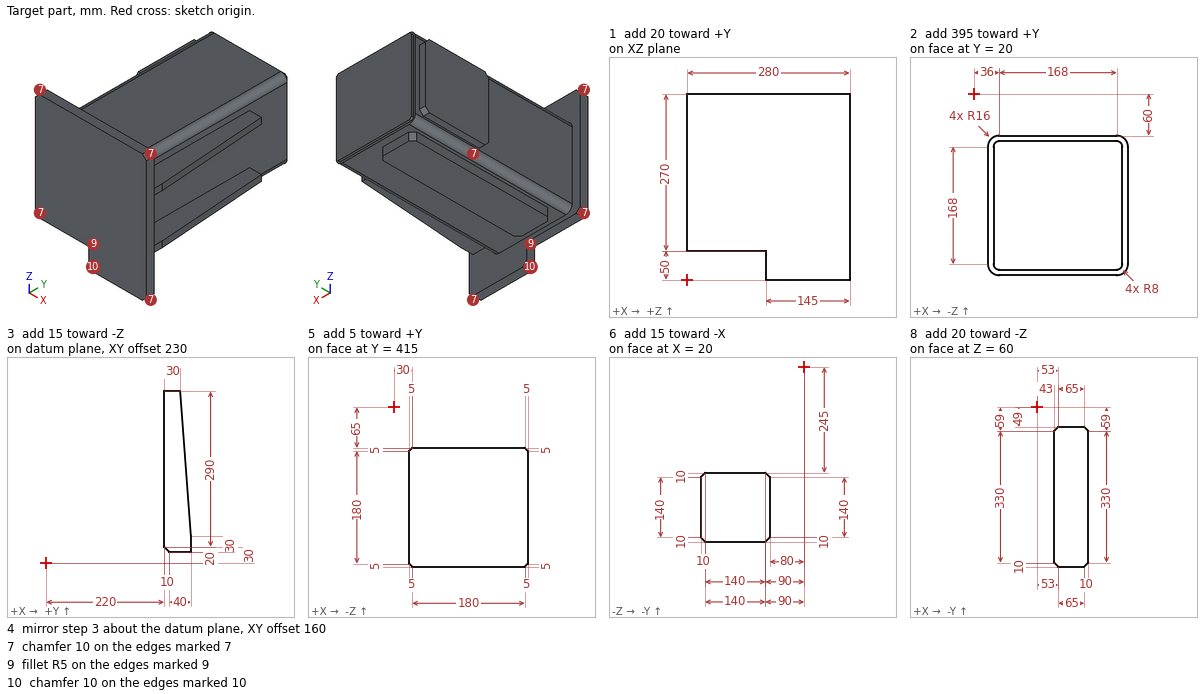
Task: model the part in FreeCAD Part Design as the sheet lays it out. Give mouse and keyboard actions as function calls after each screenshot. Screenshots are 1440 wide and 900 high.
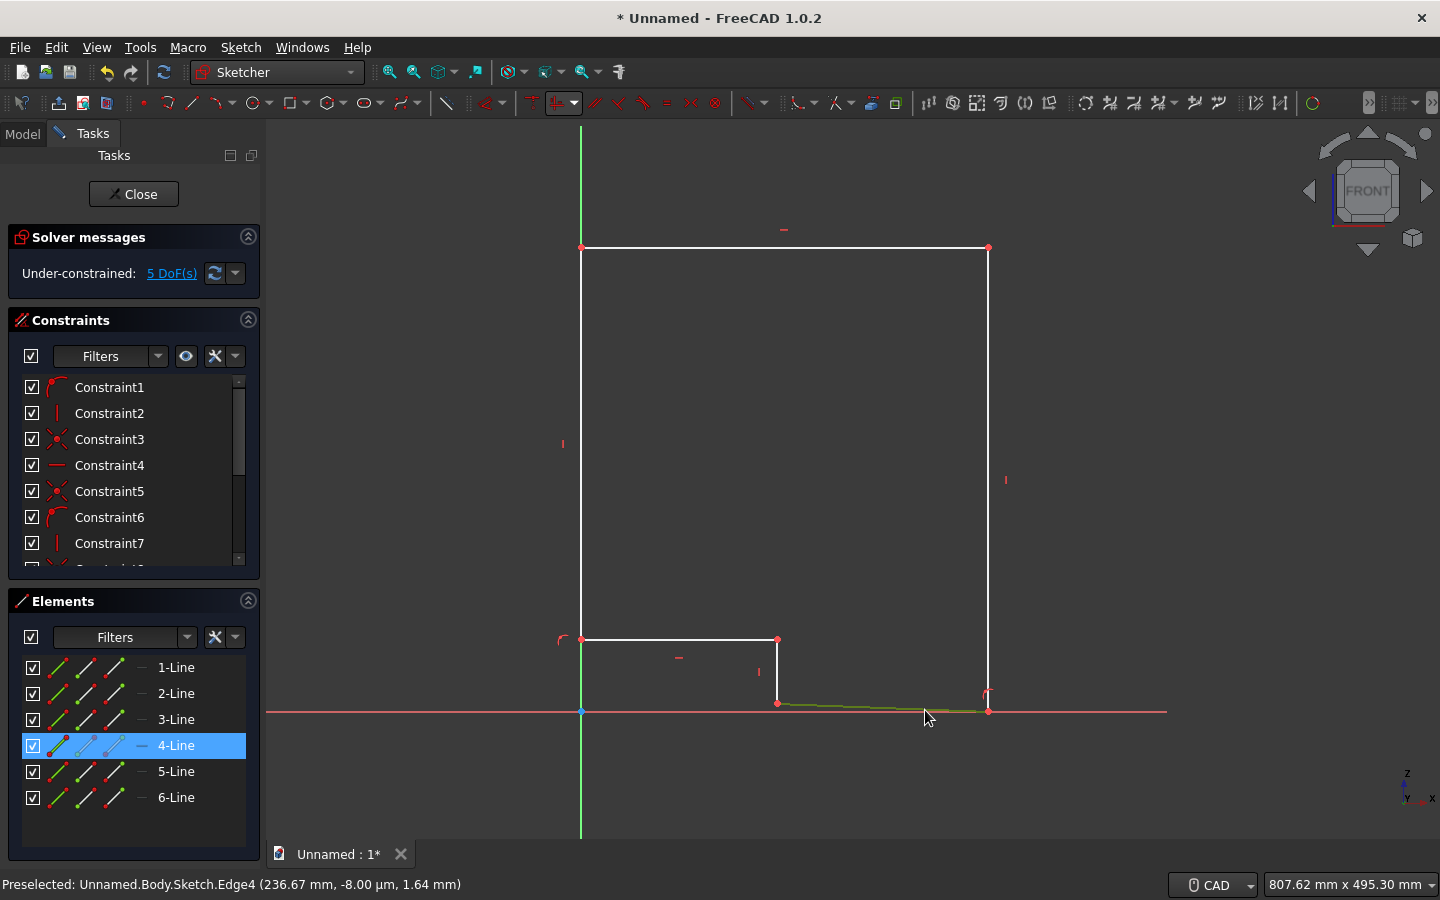
key(h)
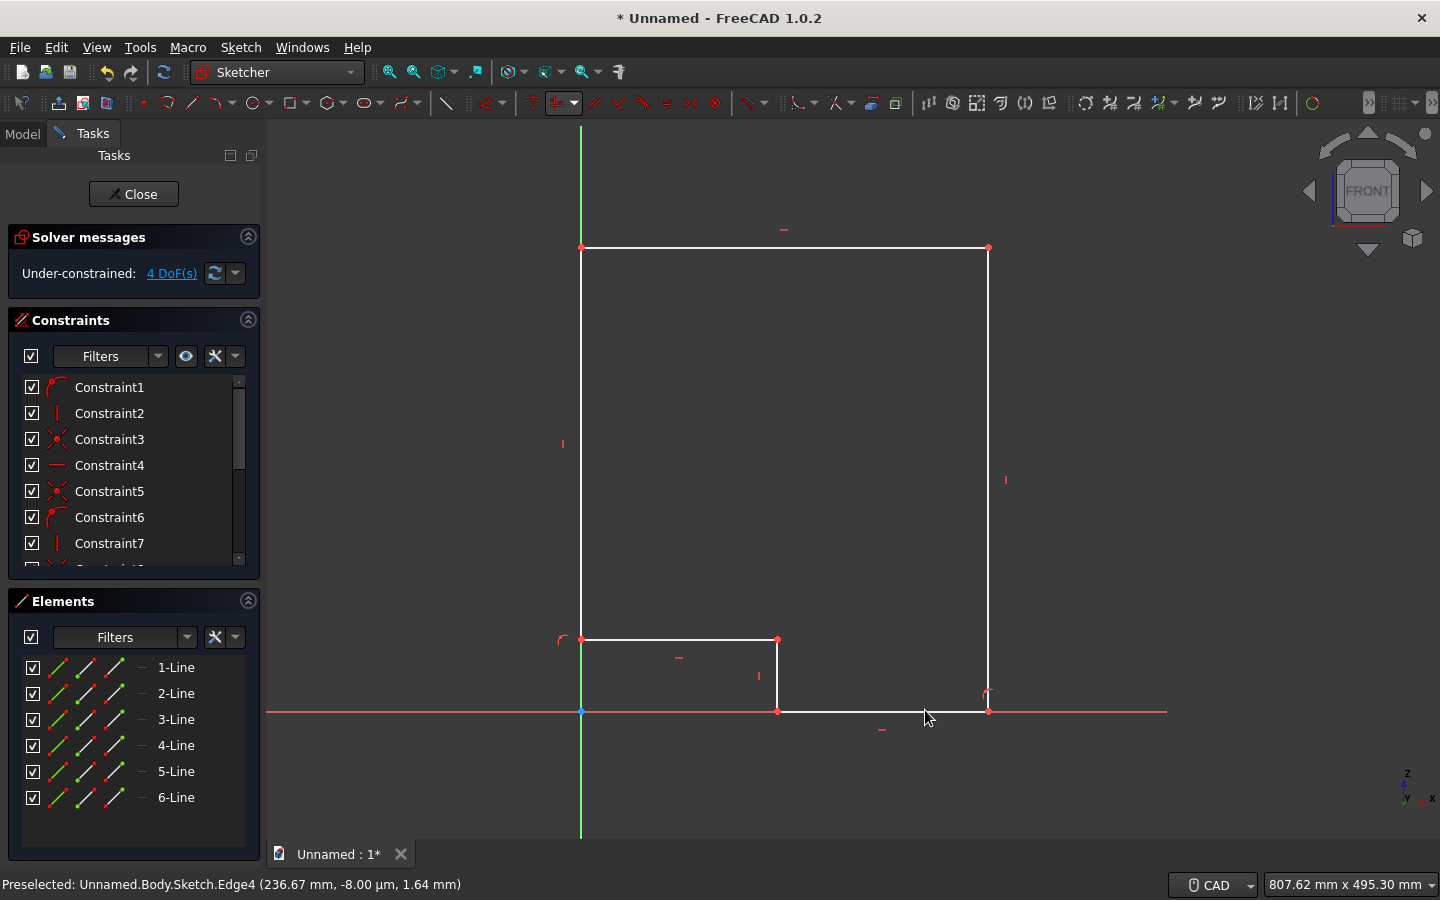
click(486, 104)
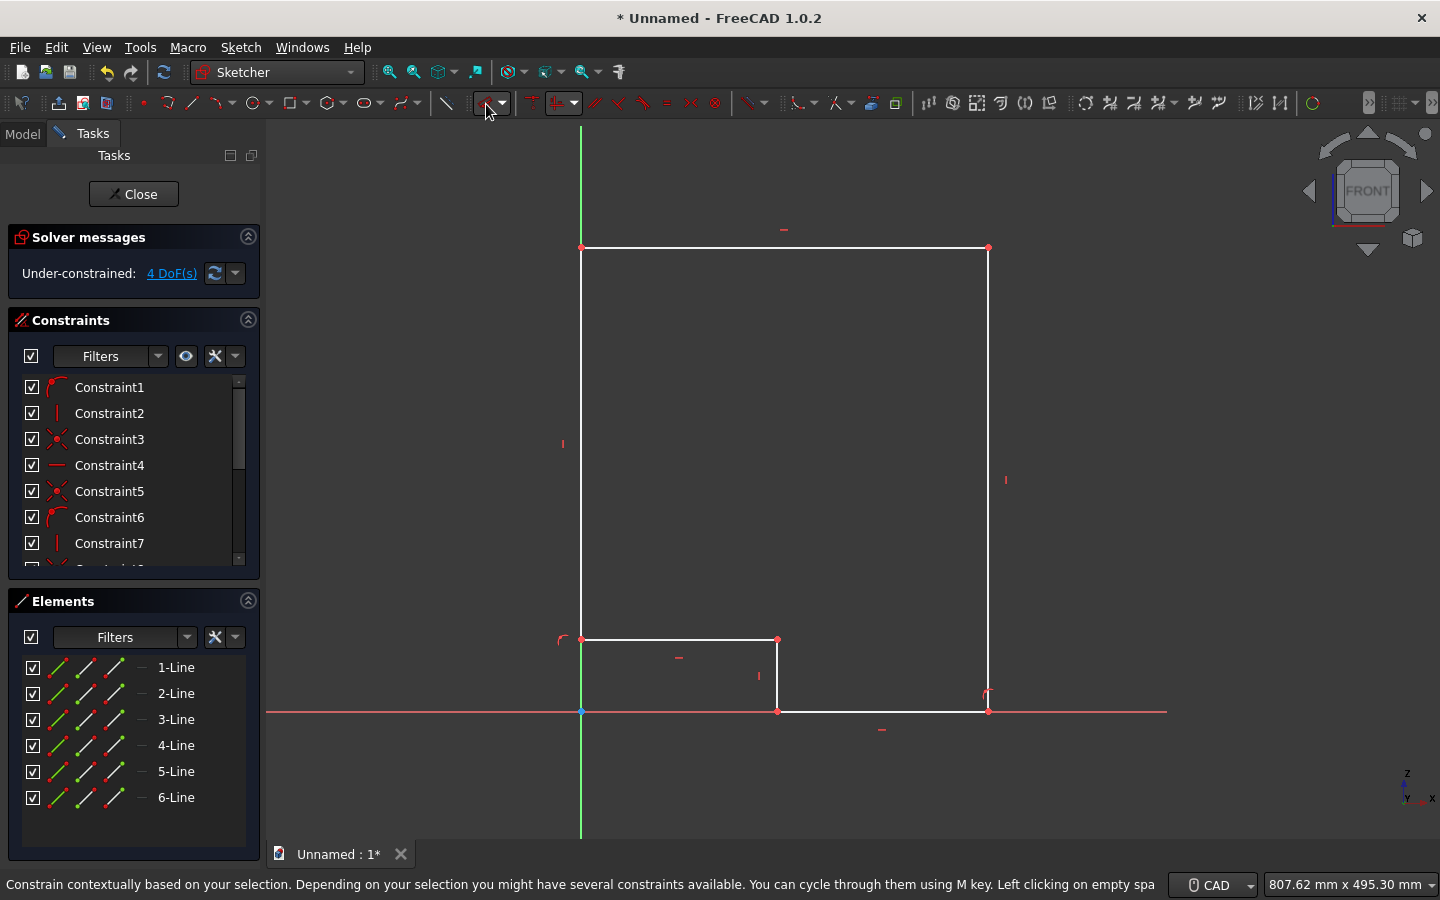
click(777, 690)
click(743, 676)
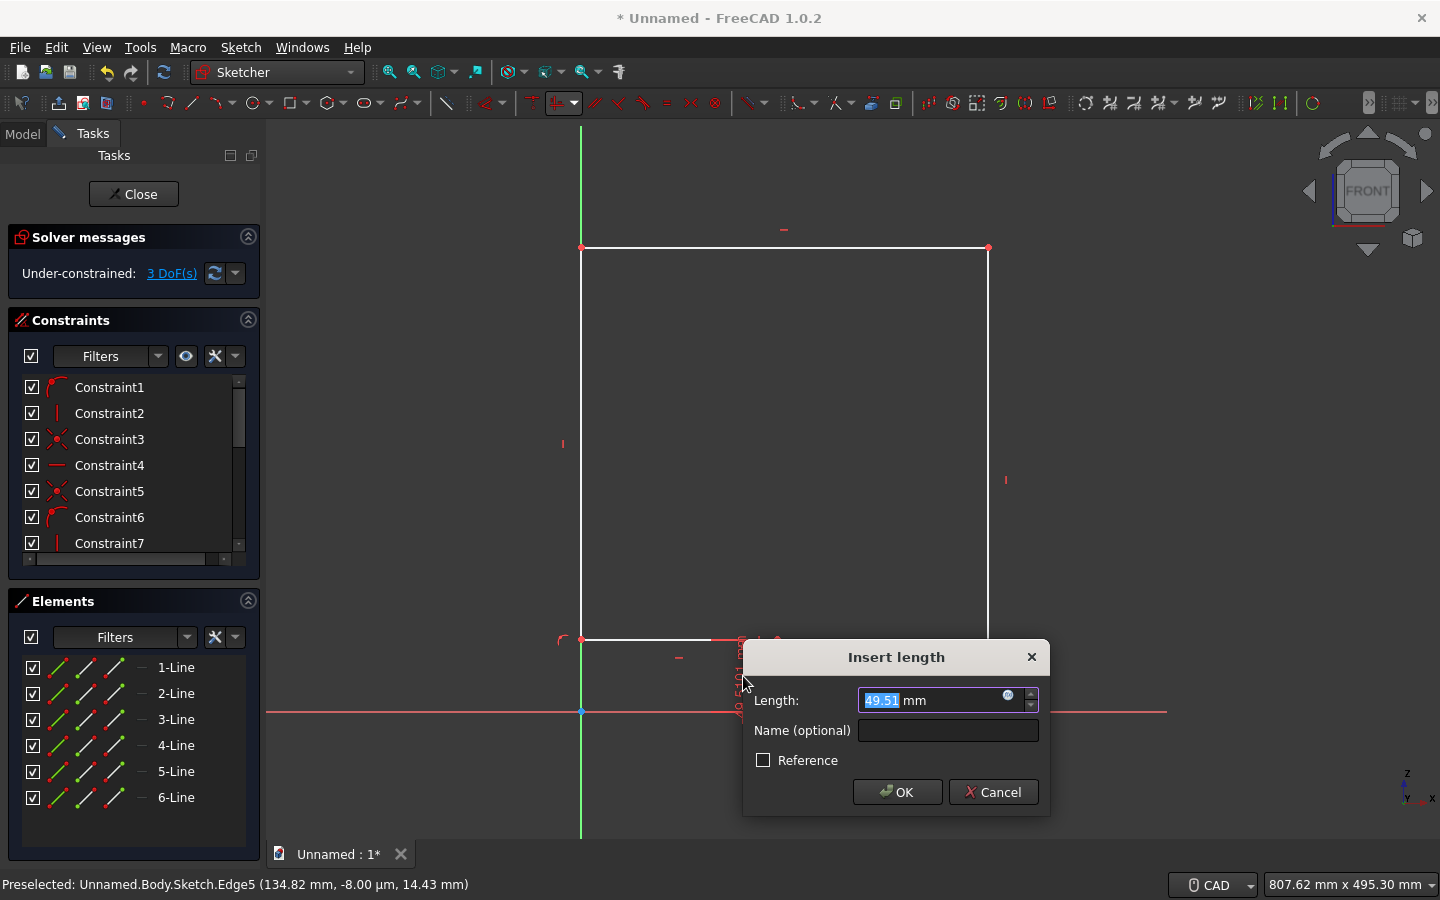
text(50)
key(Return)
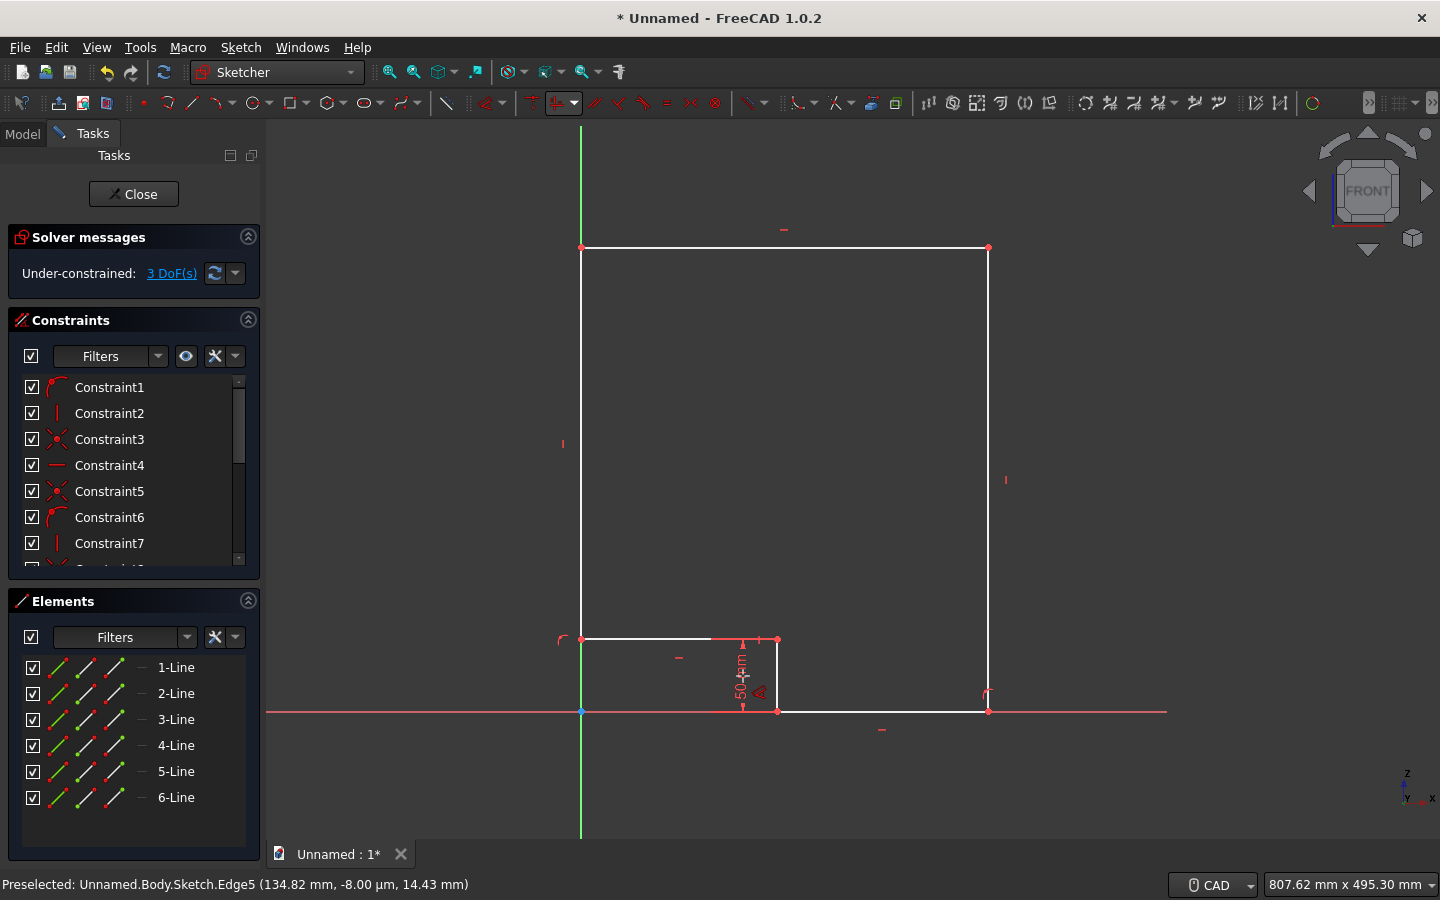
click(581, 522)
click(547, 444)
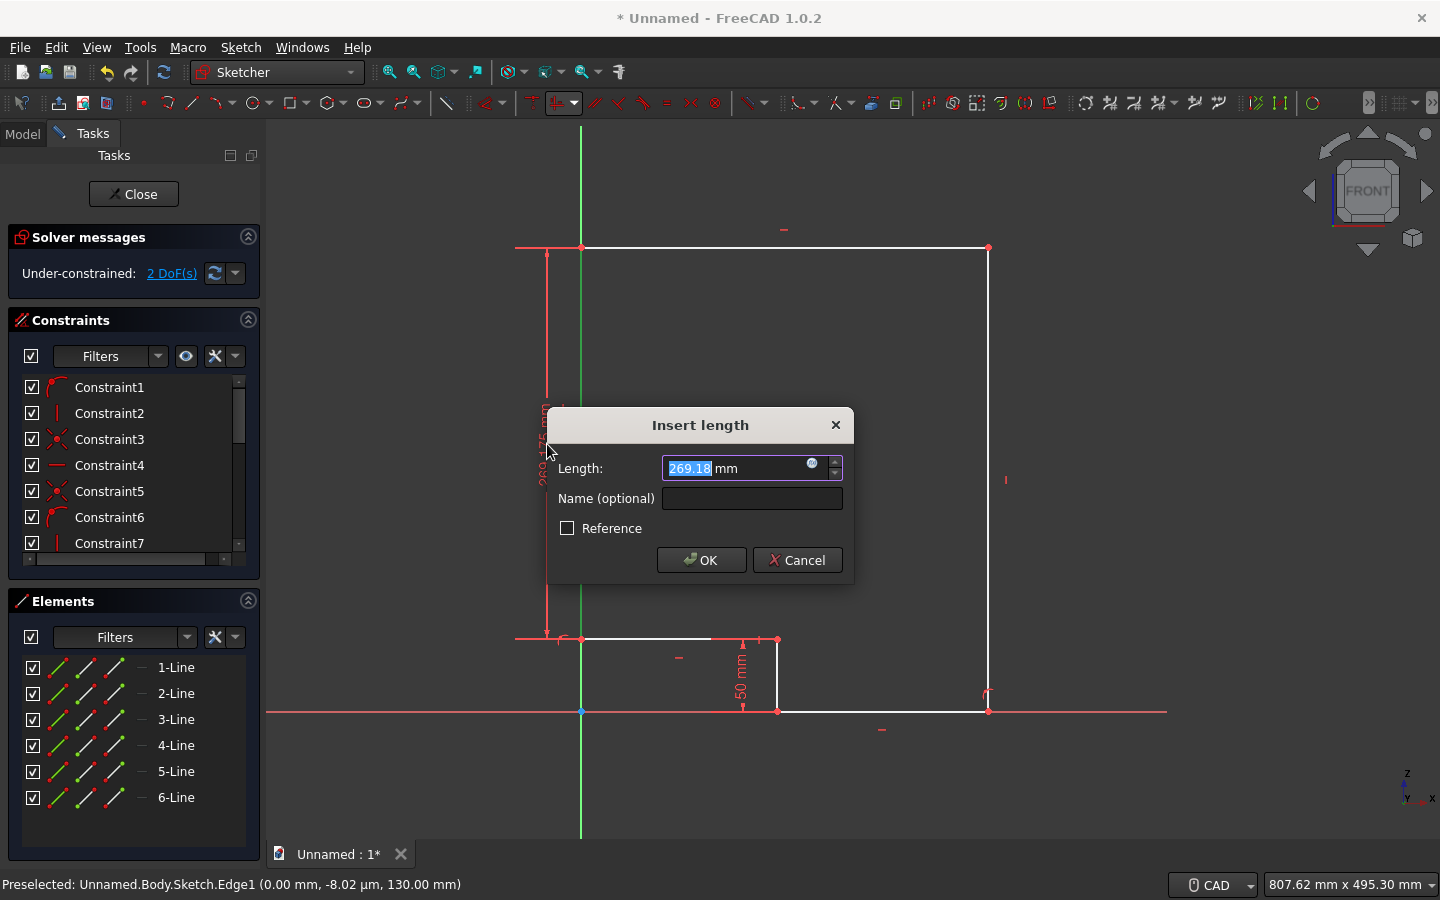
text(270)
key(Return)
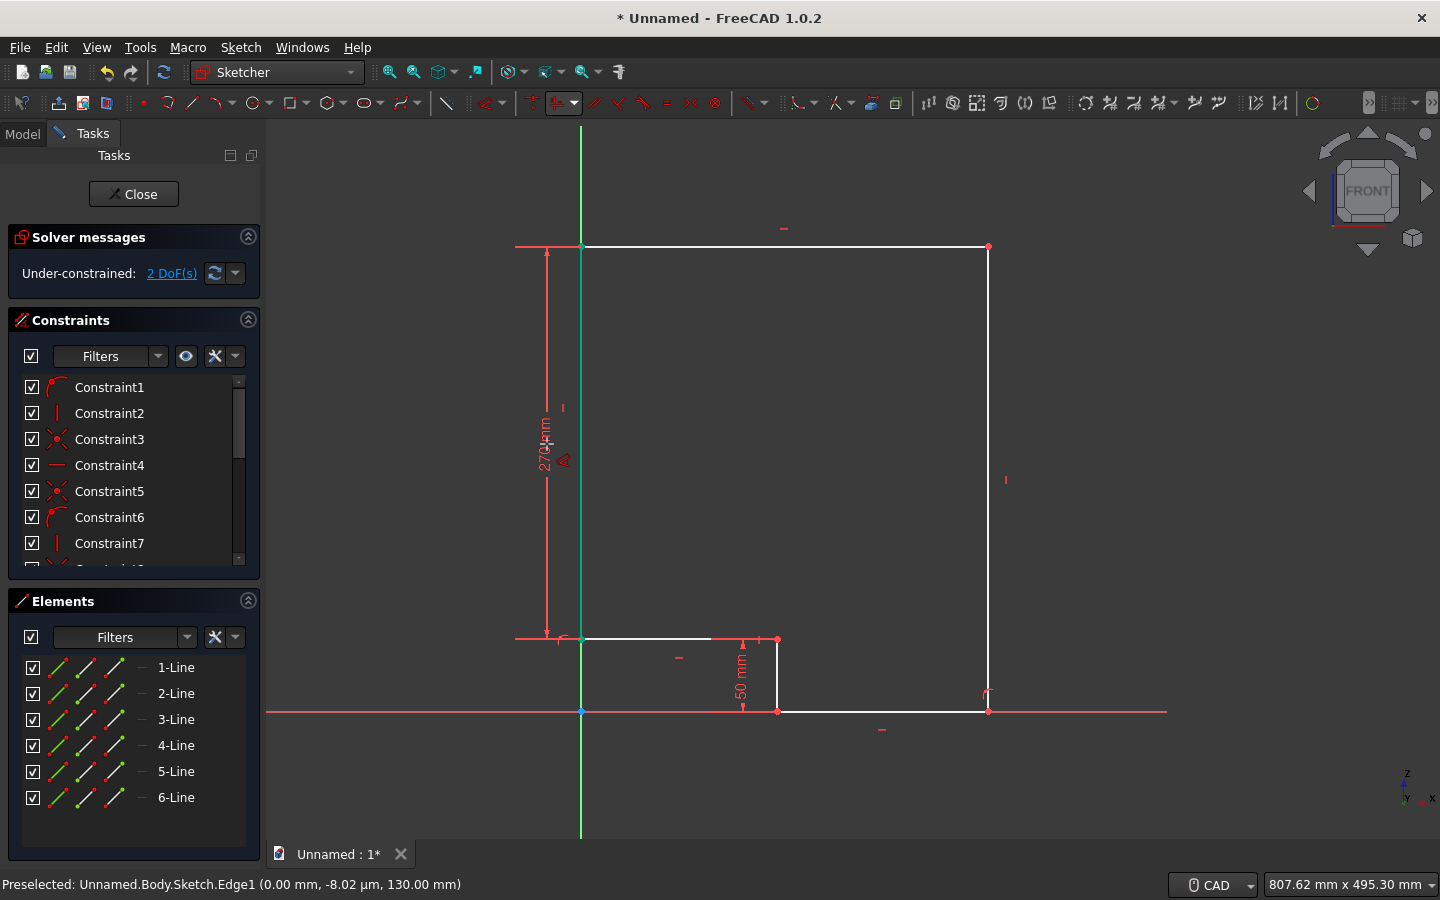
click(703, 247)
click(785, 213)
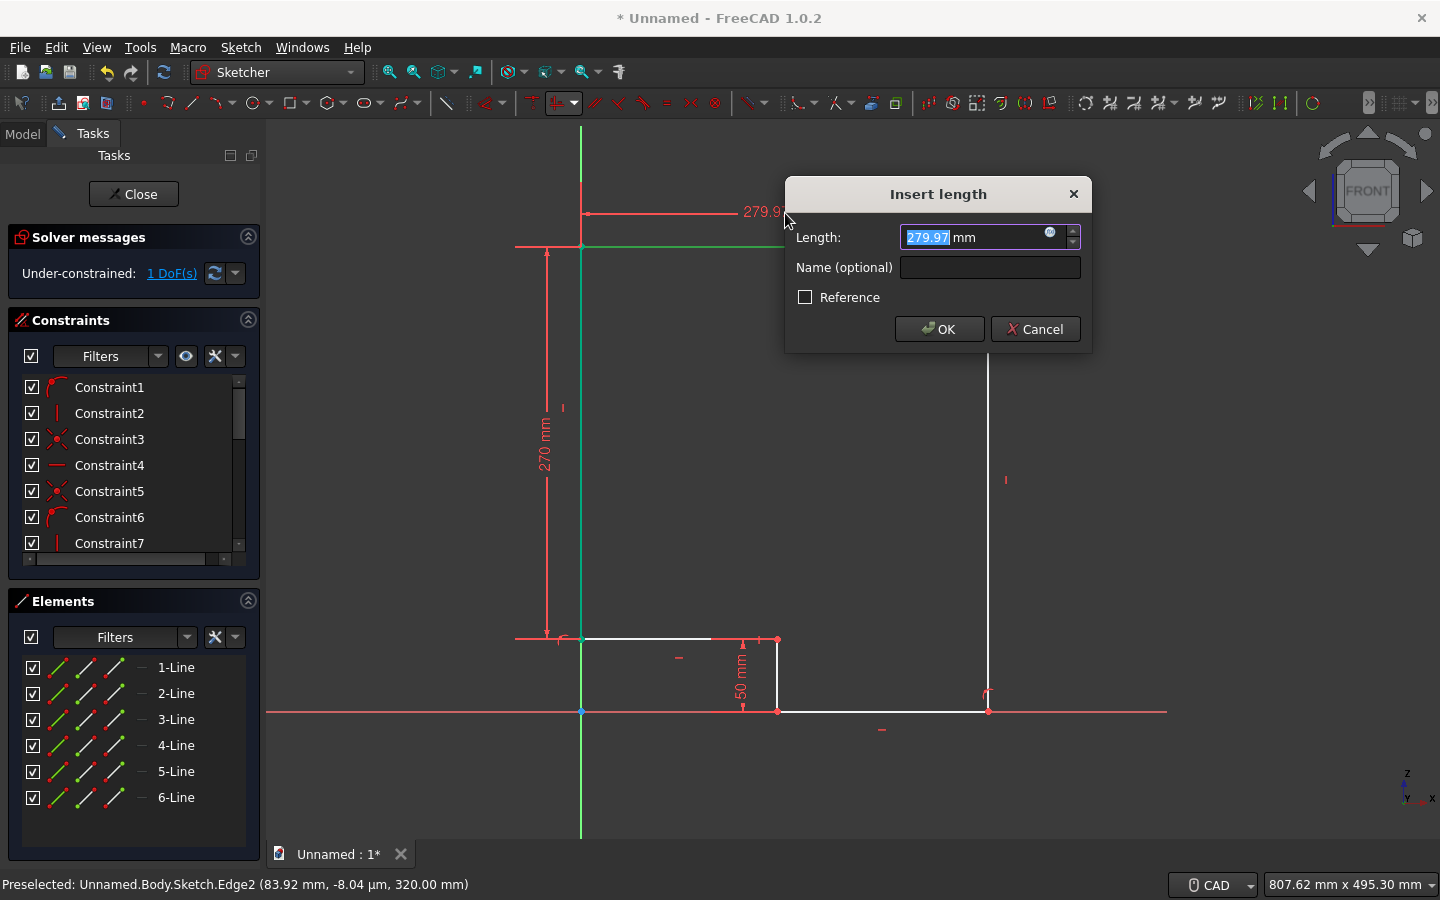
text(280)
key(Return)